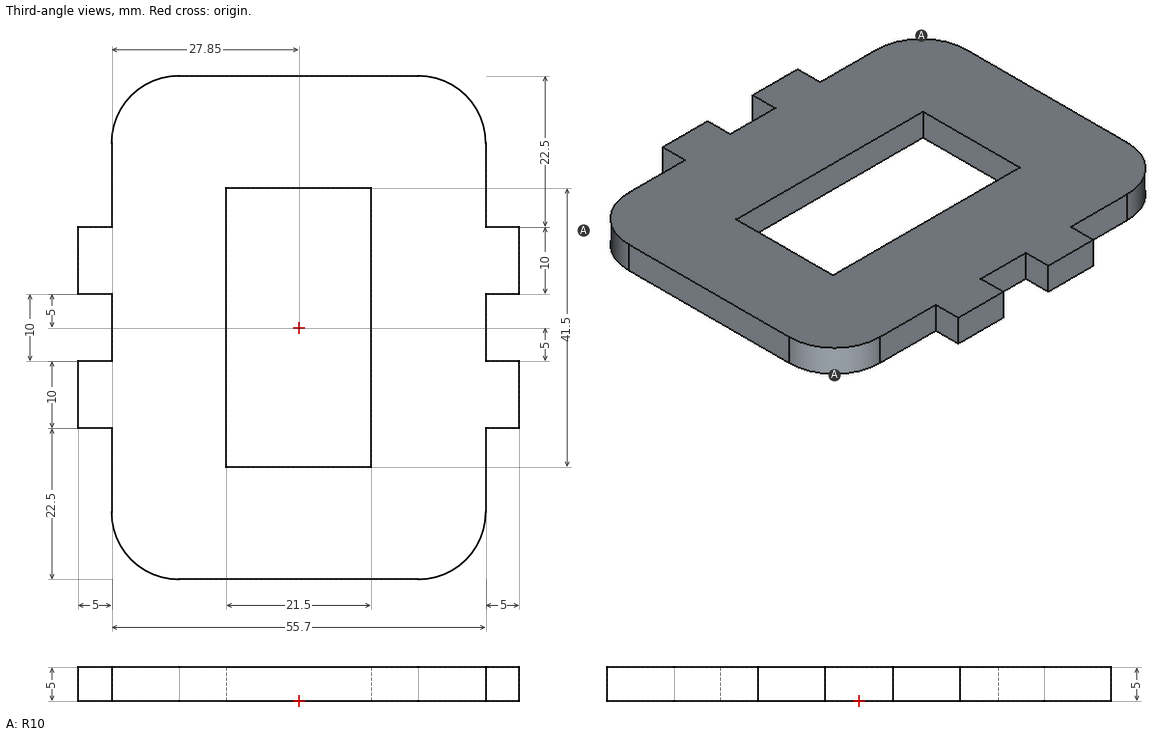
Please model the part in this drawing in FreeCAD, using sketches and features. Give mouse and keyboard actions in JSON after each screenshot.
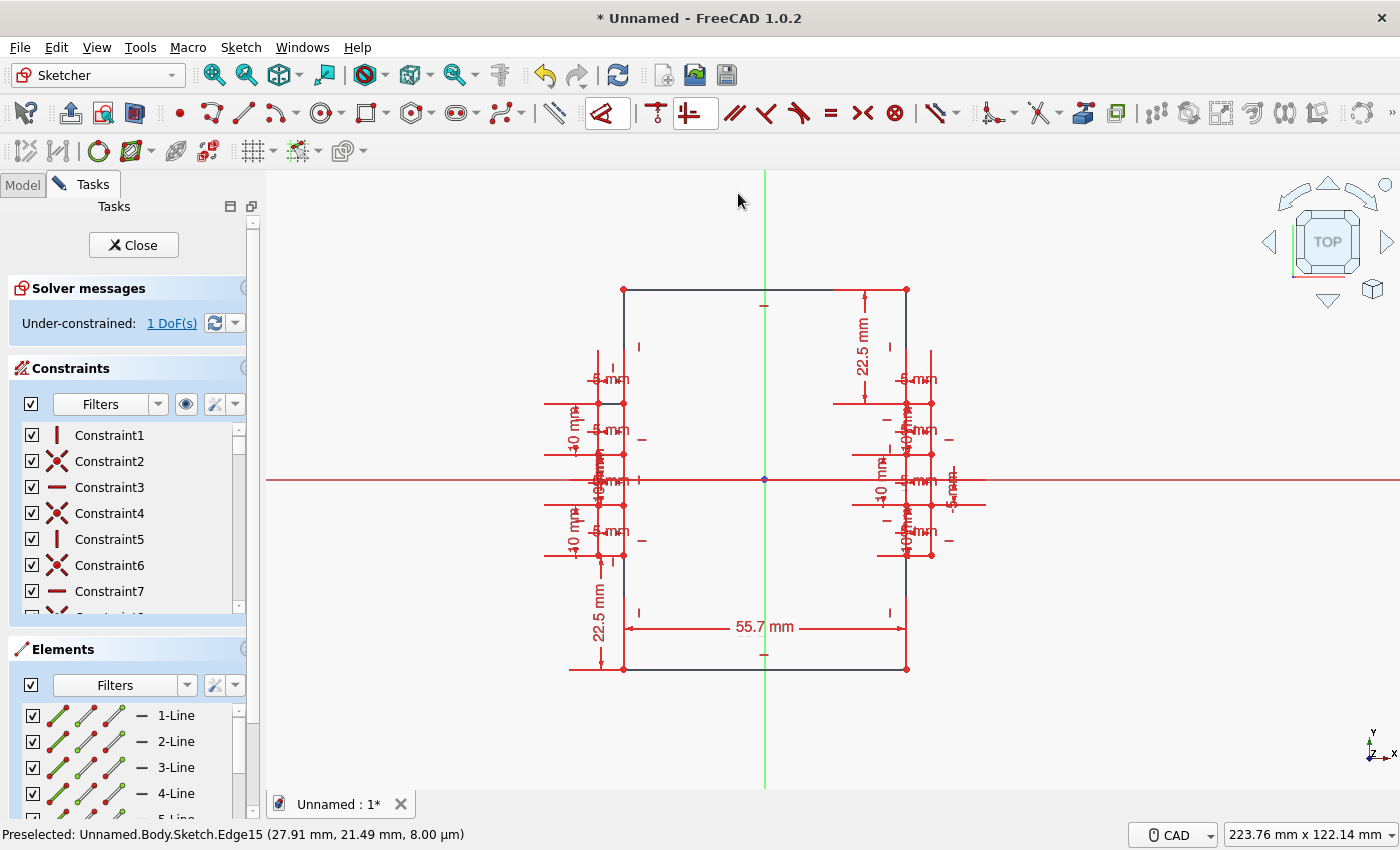
{"action": "left_click", "coordinate": [624, 455]}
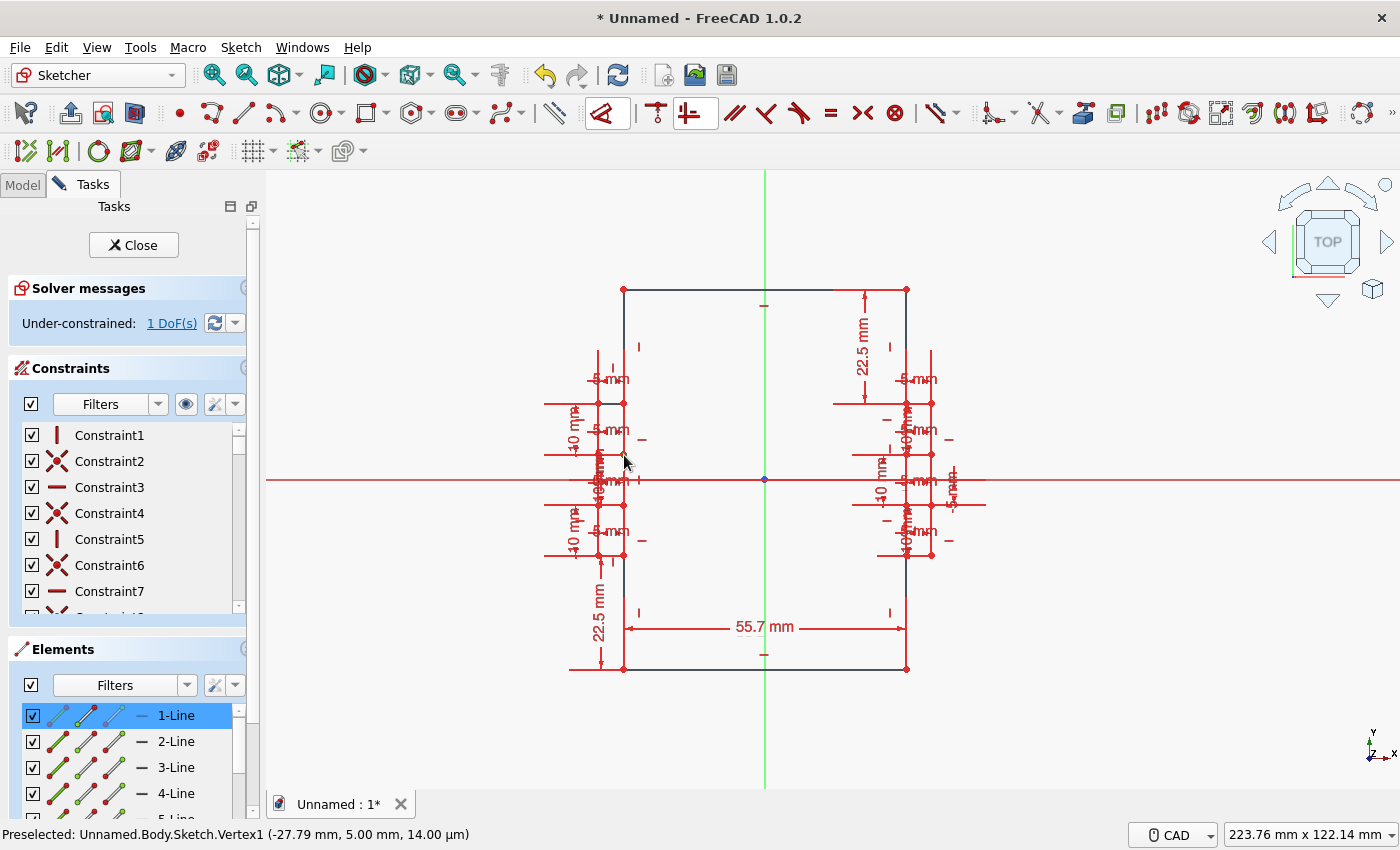
{"action": "key", "text": "l"}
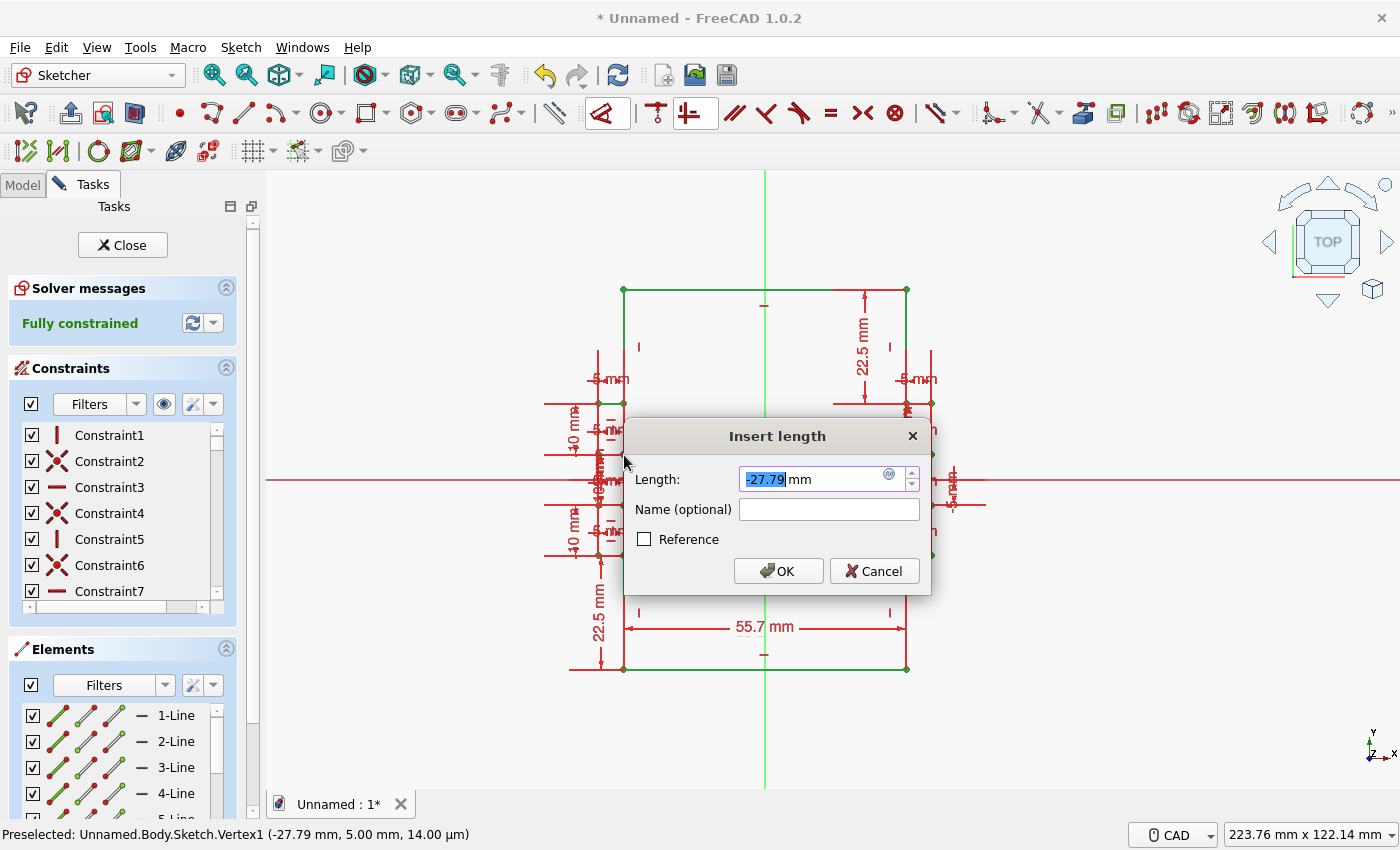
{"action": "type", "text": "-27.85"}
{"action": "key", "text": "Return"}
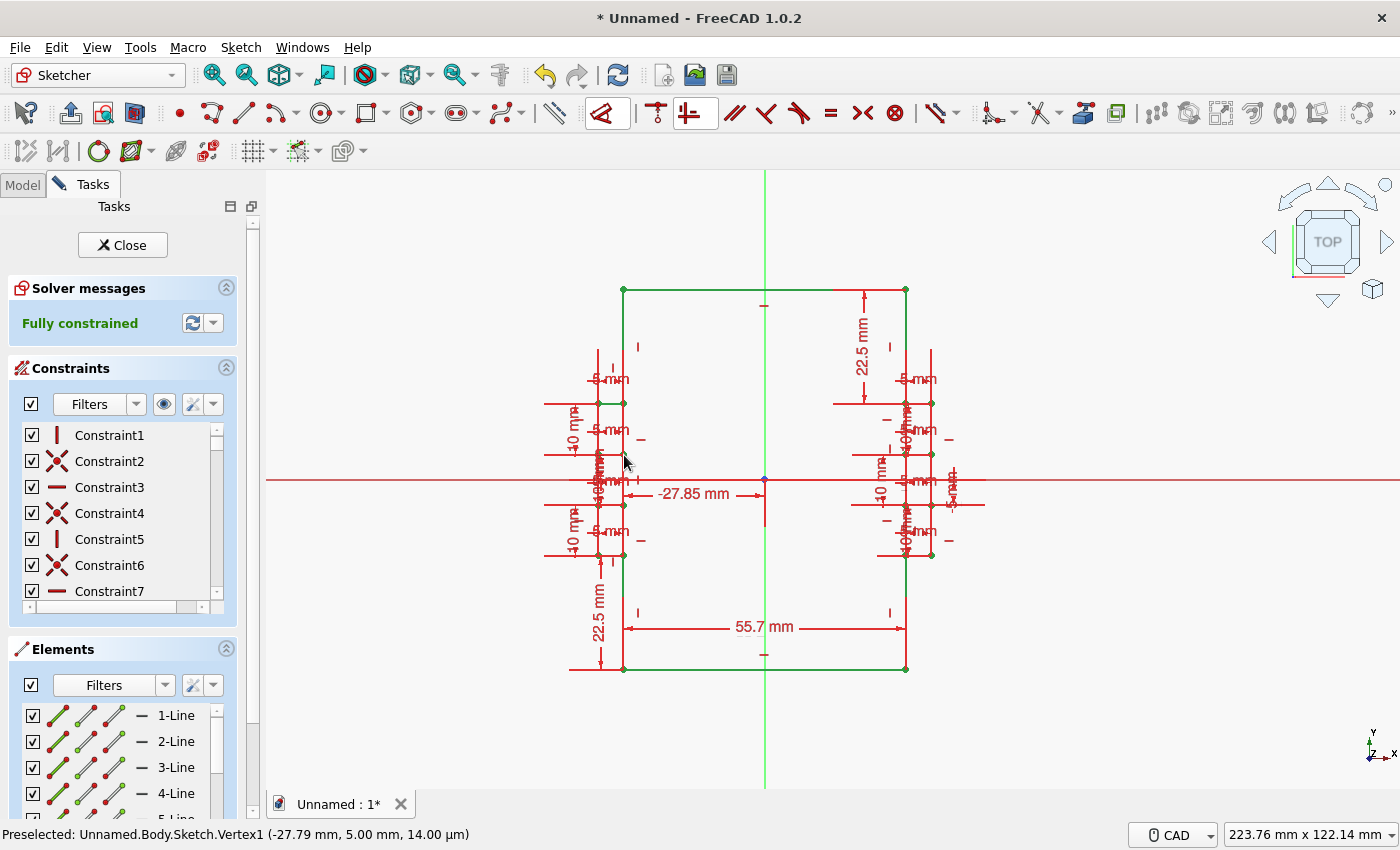
{"action": "left_click", "coordinate": [123, 245]}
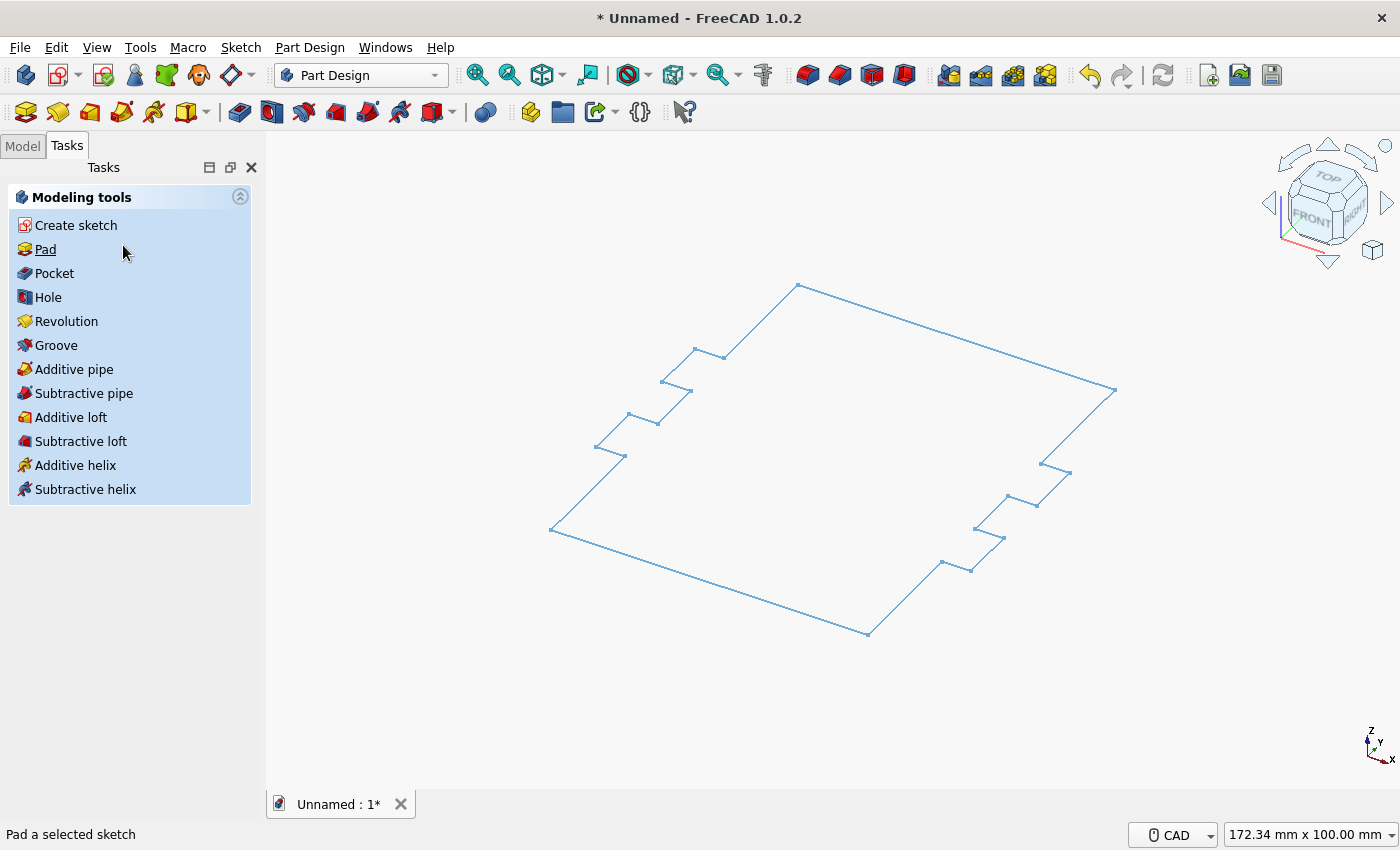
{"action": "left_click", "coordinate": [26, 112]}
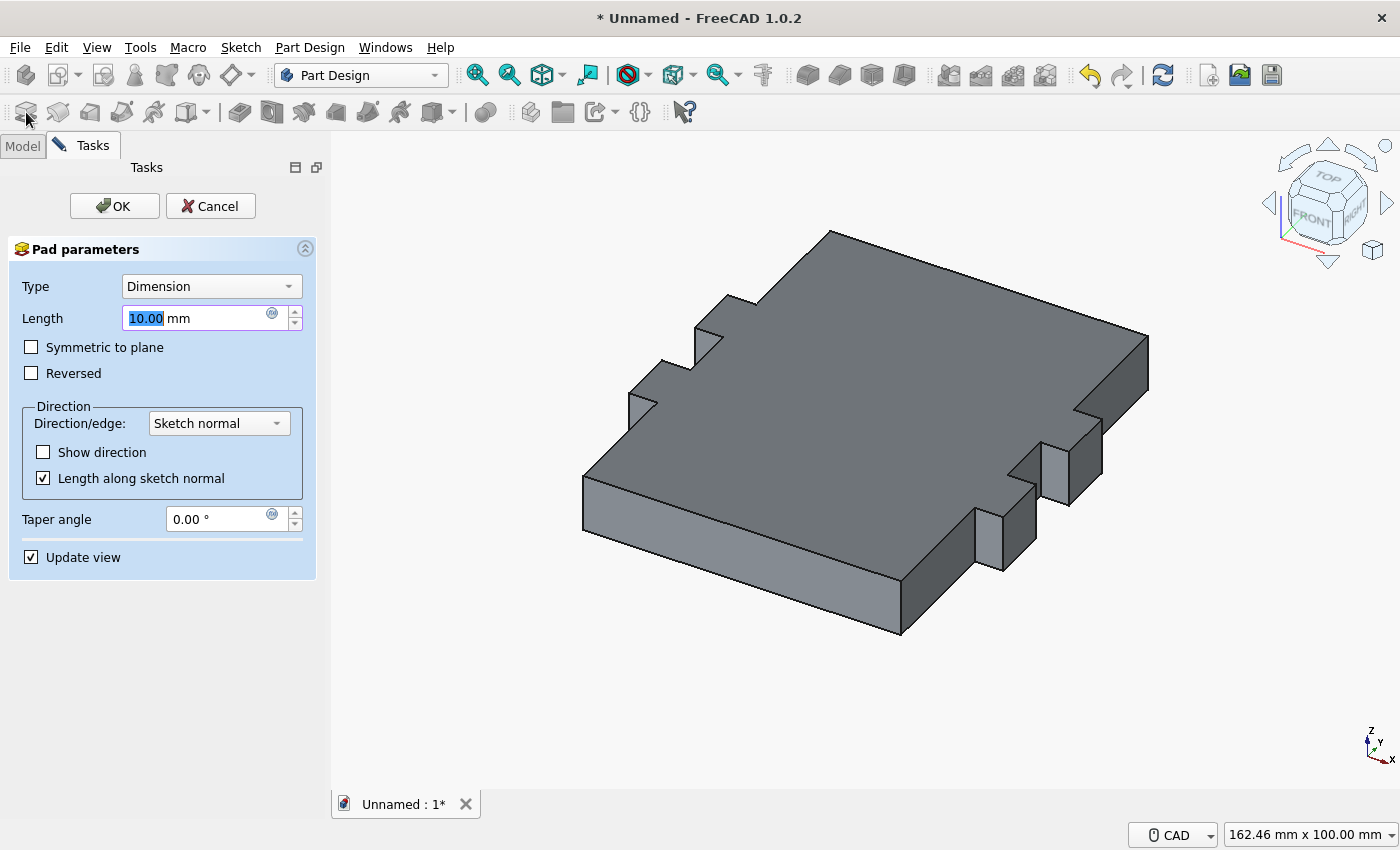
{"action": "type", "text": "5"}
{"action": "key", "text": "Tab"}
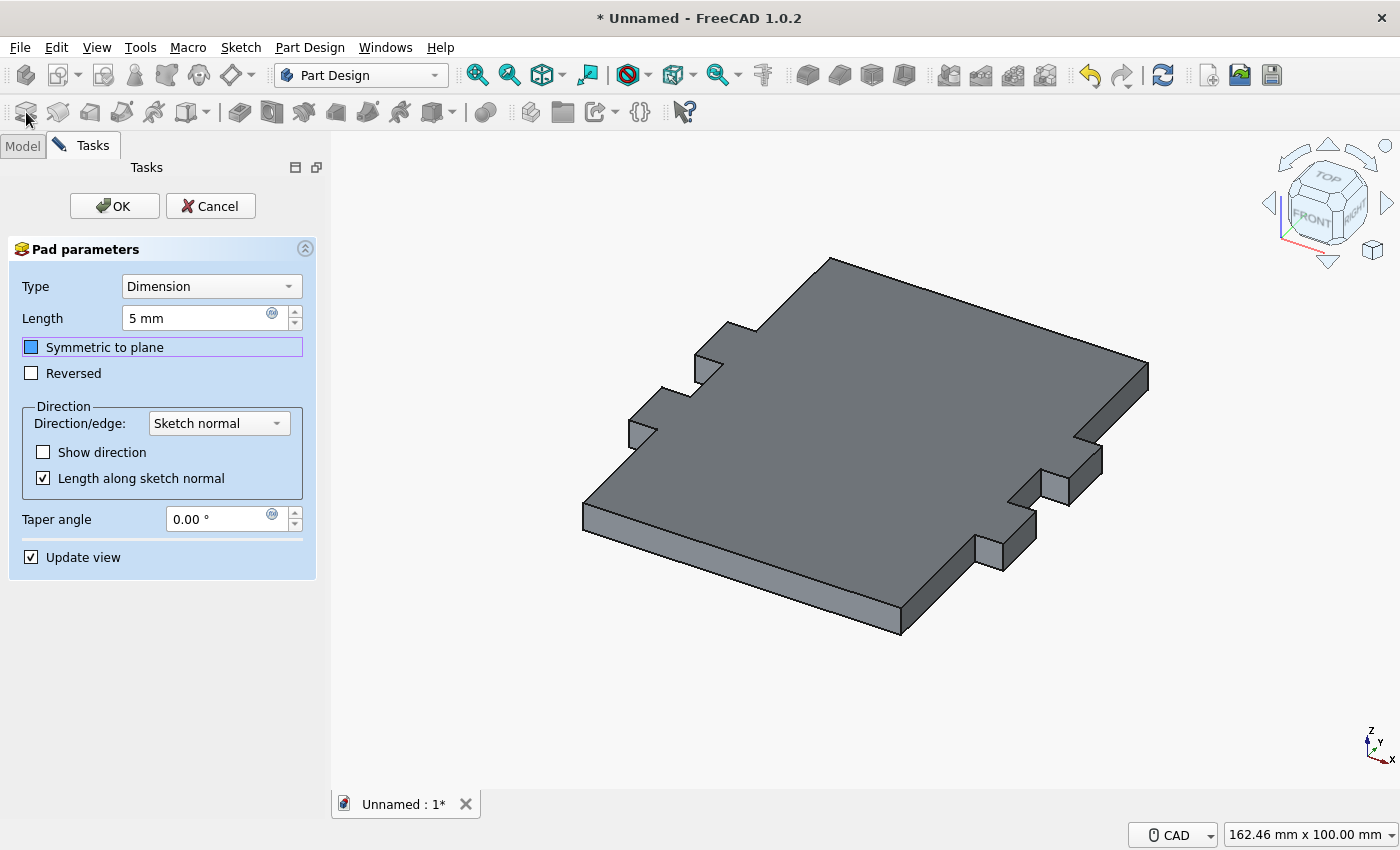
{"action": "left_click", "coordinate": [115, 206]}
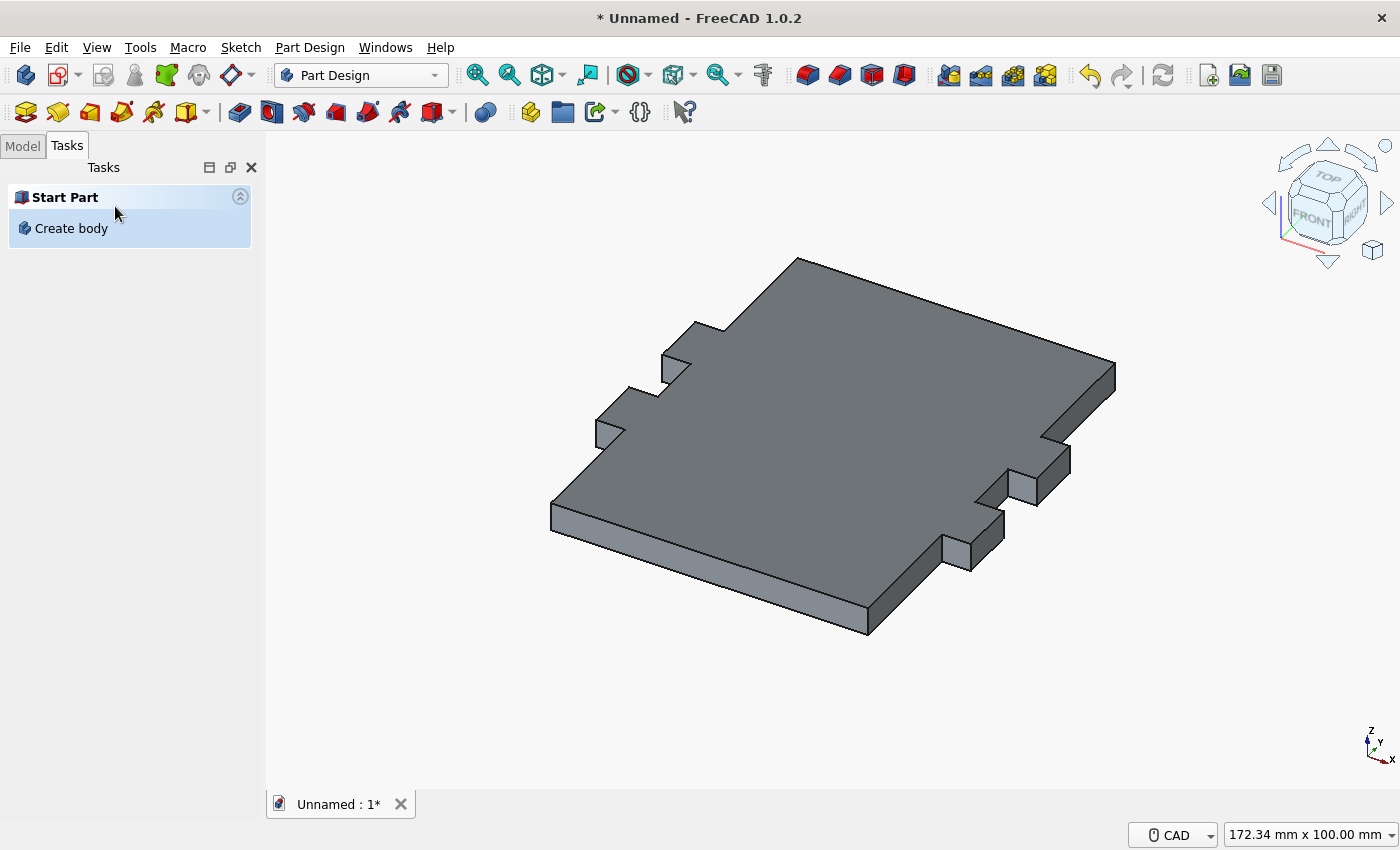
{"action": "left_click", "coordinate": [833, 432]}